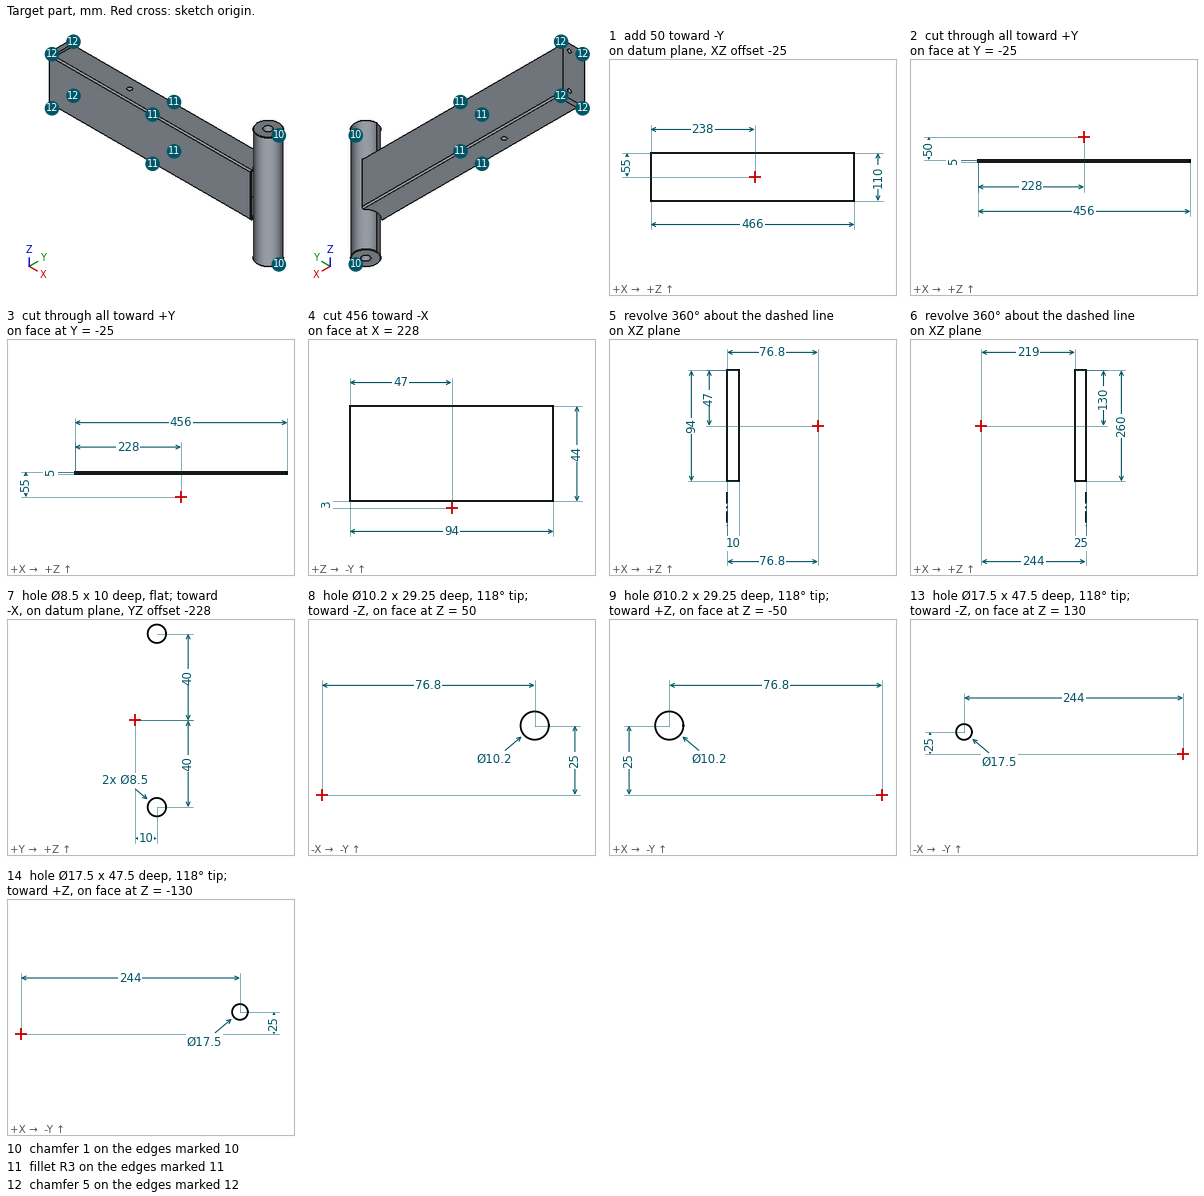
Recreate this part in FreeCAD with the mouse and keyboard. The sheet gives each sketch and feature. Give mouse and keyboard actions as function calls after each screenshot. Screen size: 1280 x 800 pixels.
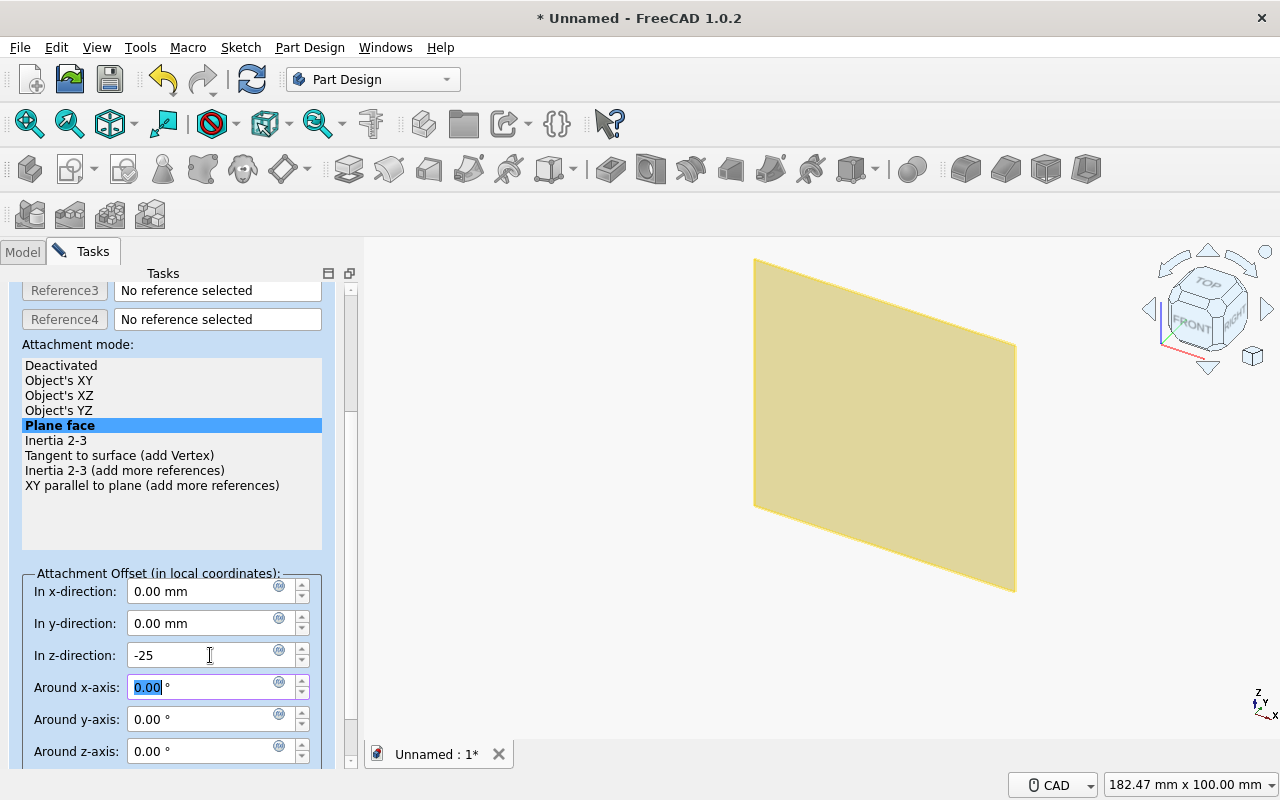
scroll(351, 526, up, 4)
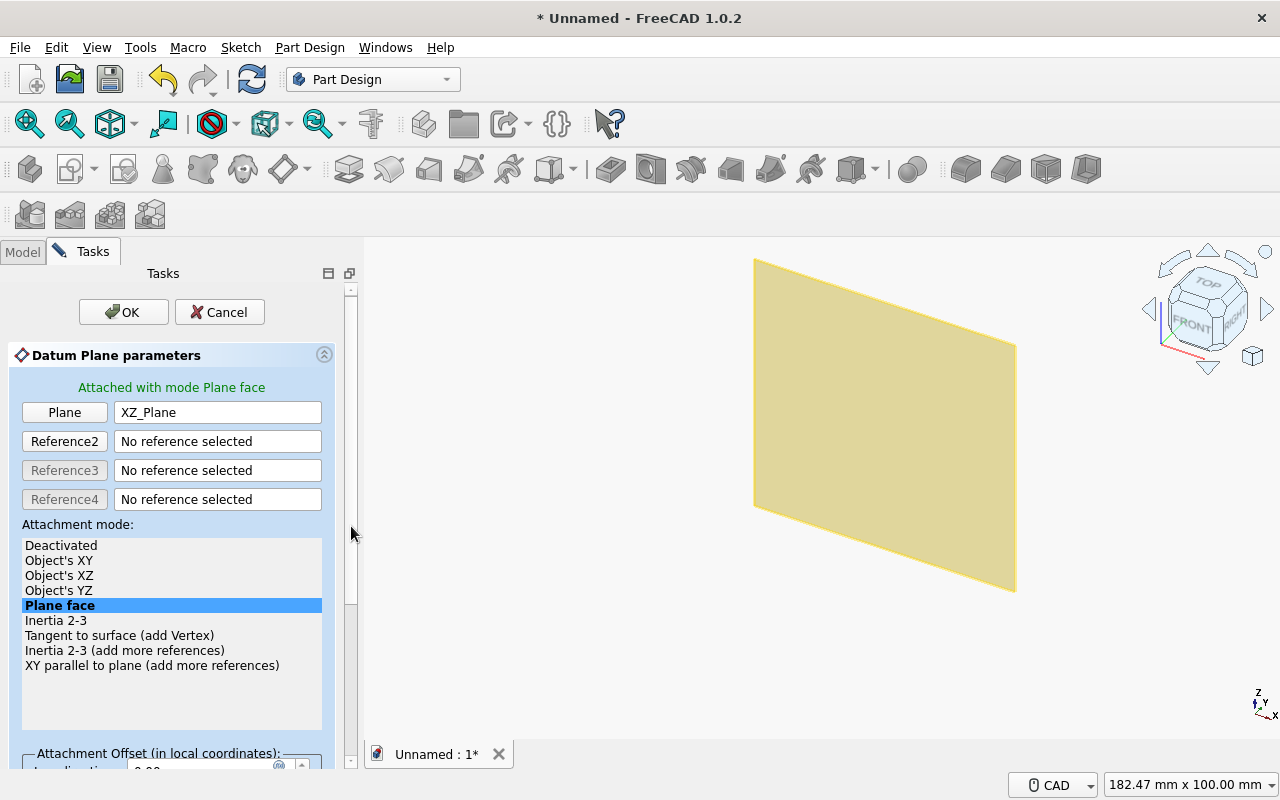
click(124, 312)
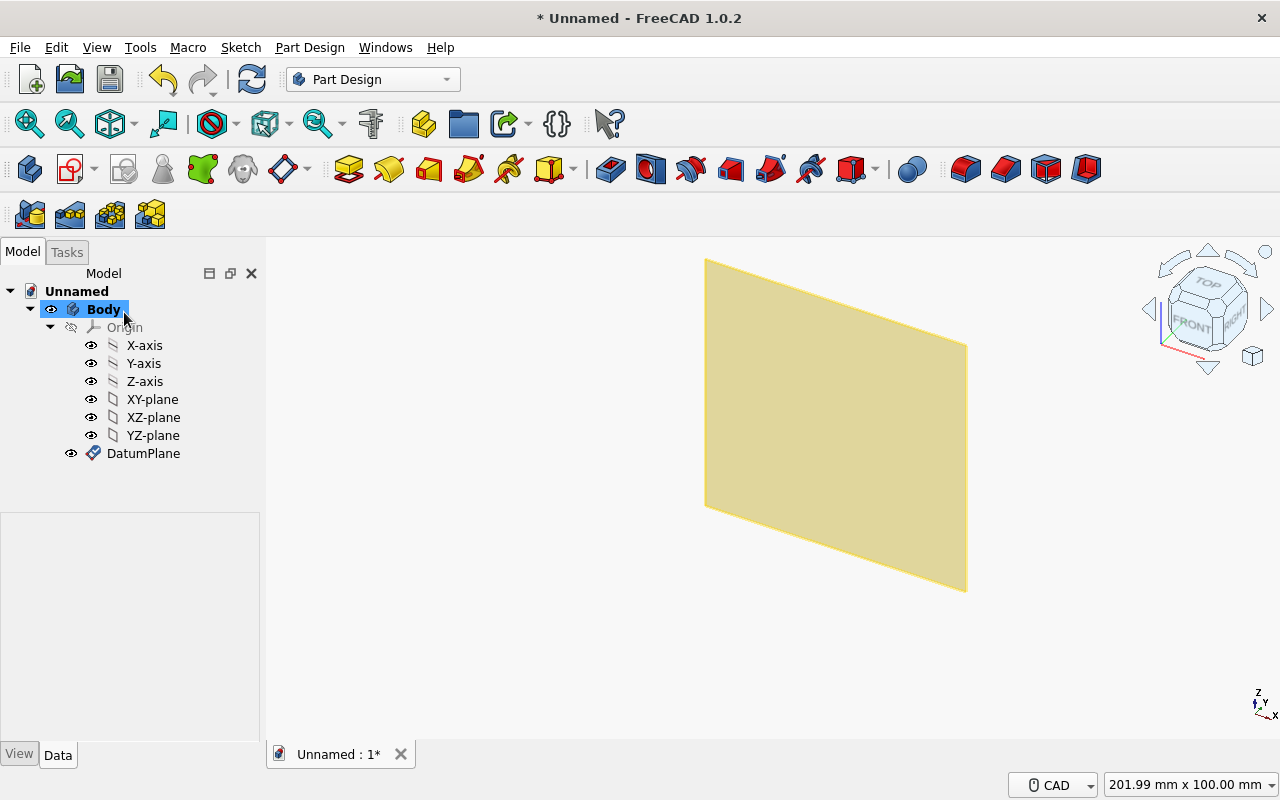
click(116, 453)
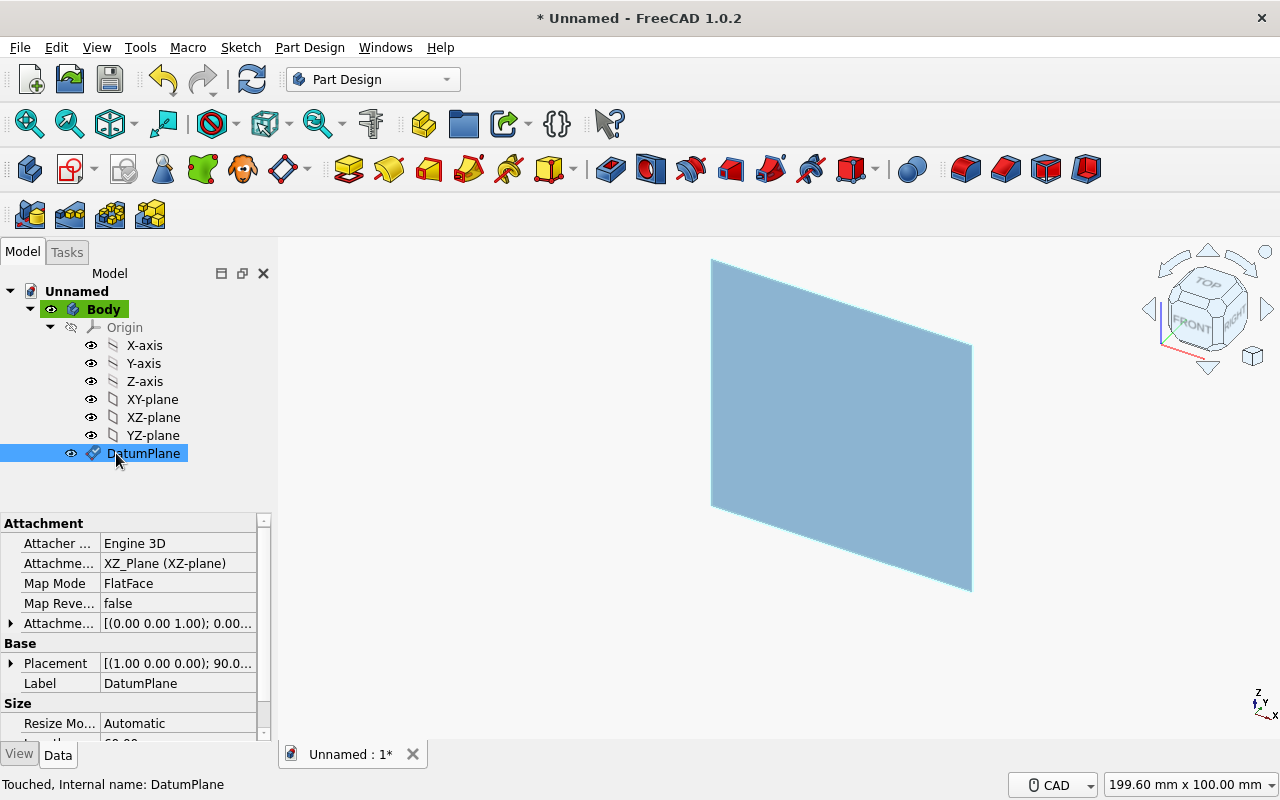
click(70, 170)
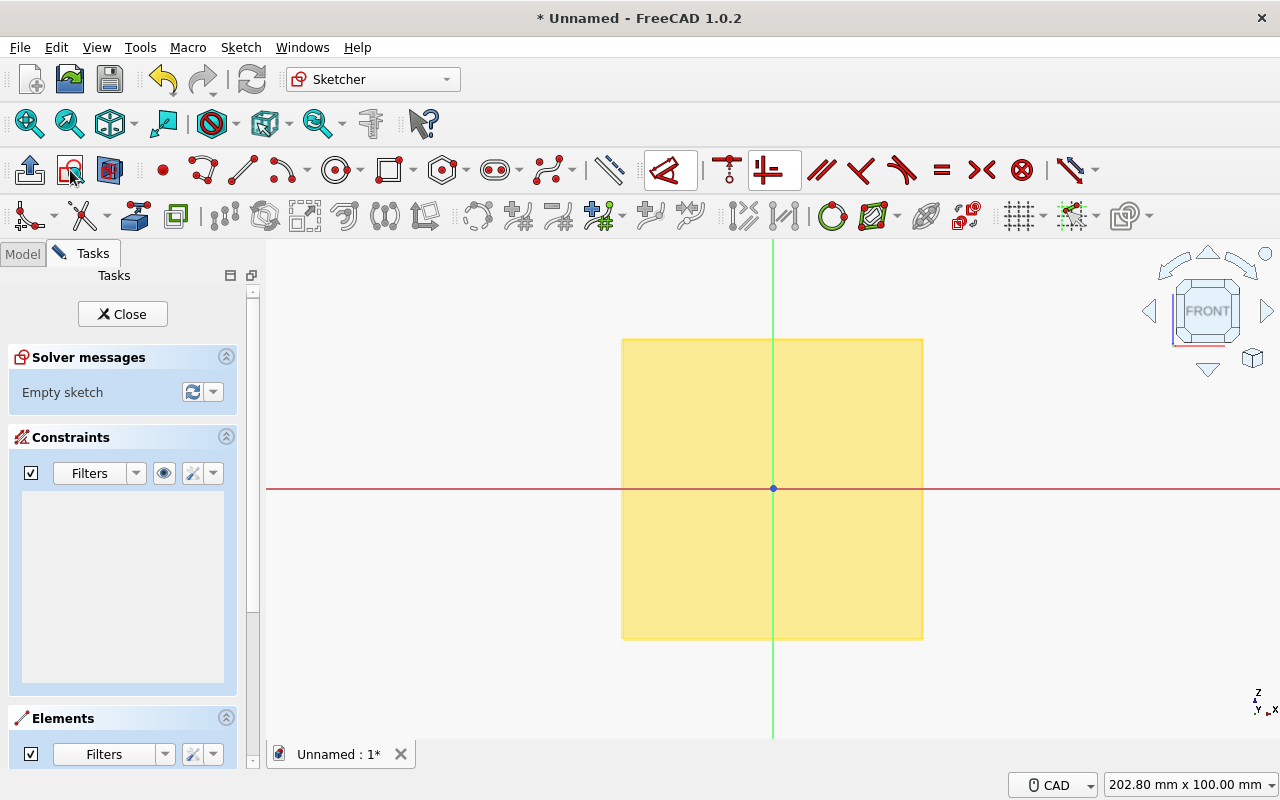
scroll(690, 489, down, 7)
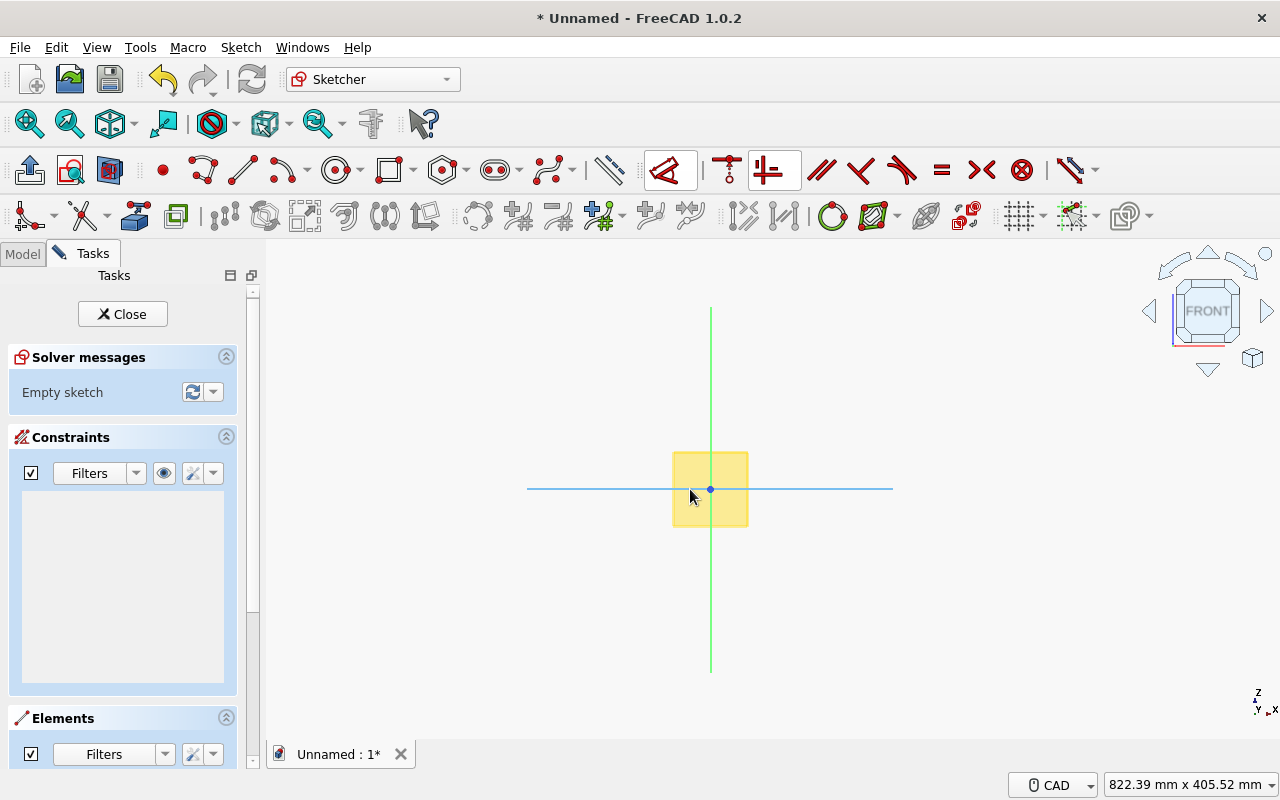
click(390, 170)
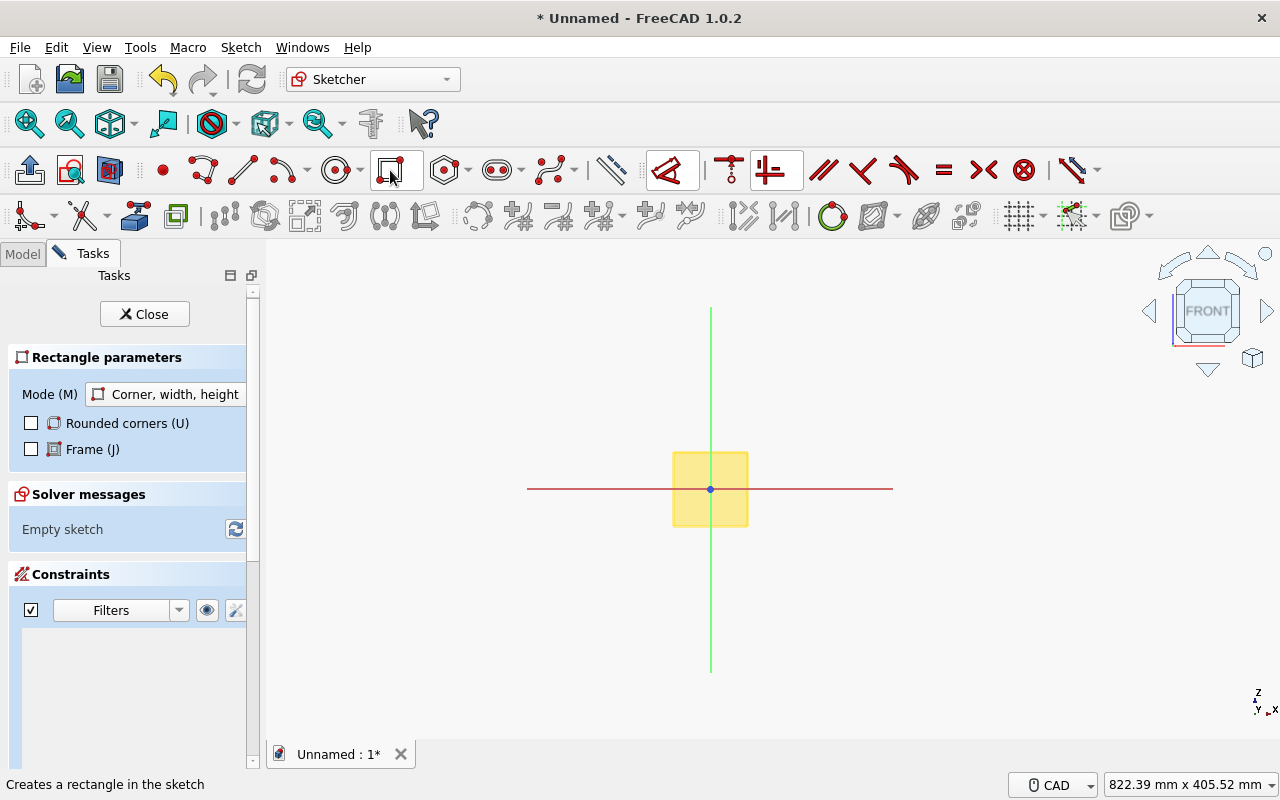
click(417, 422)
move(992, 557)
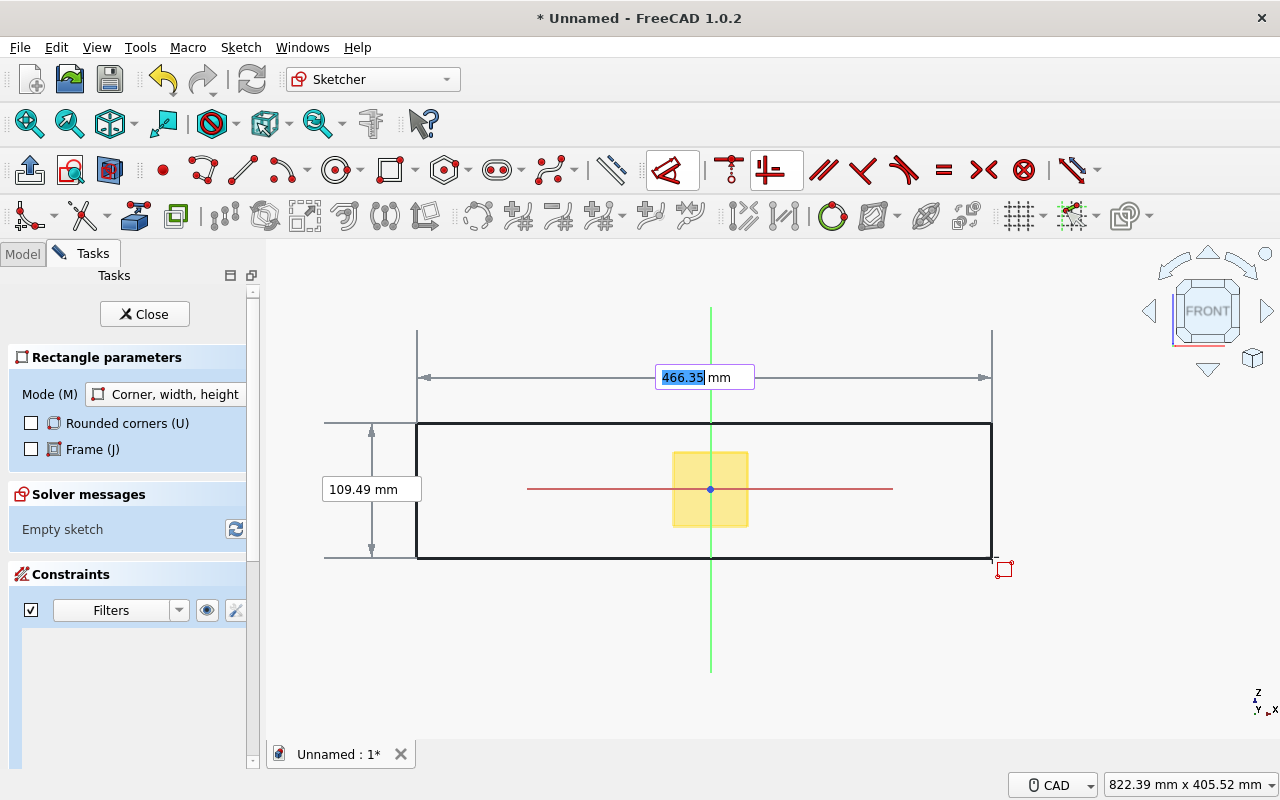
text(466)
key(Tab)
text(110)
key(Return)
key(Escape)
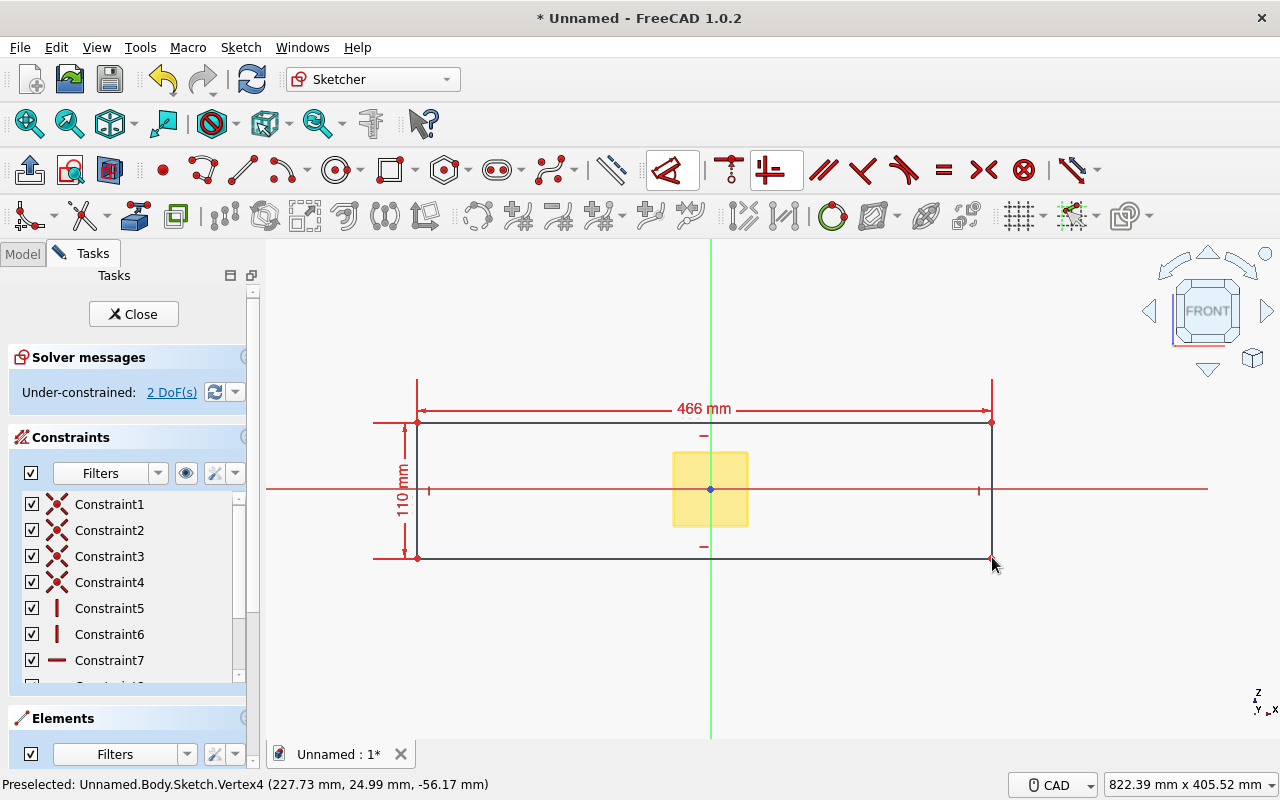
click(666, 170)